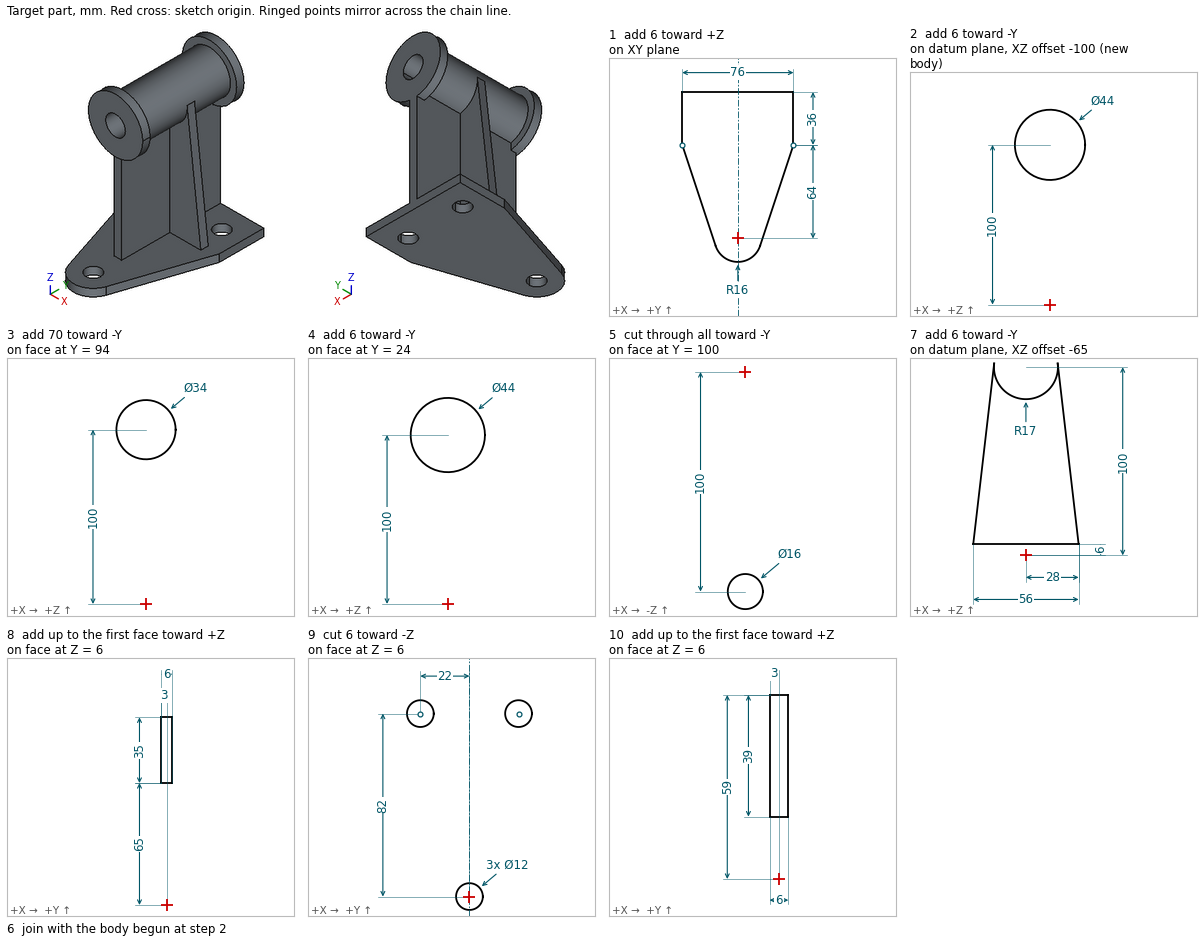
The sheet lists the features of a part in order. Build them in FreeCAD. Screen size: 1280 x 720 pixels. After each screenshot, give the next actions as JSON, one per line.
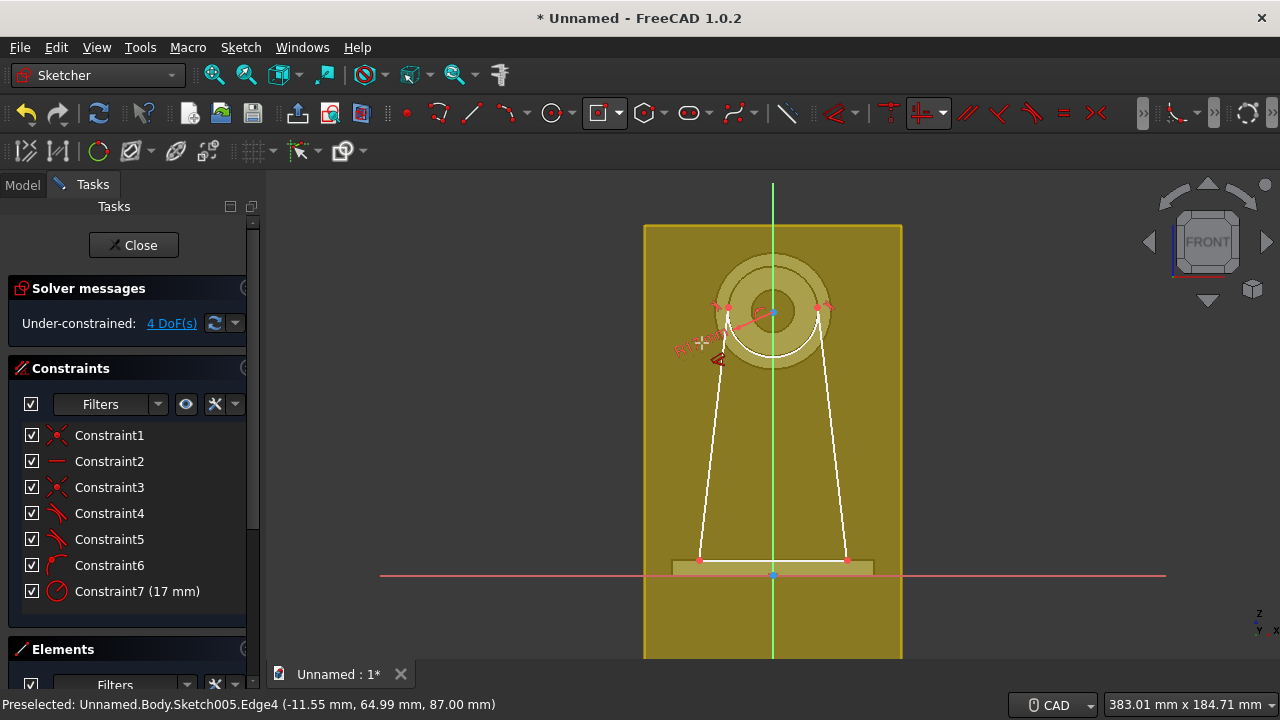
{"action": "left_click", "coordinate": [803, 561]}
{"action": "left_click", "coordinate": [739, 595]}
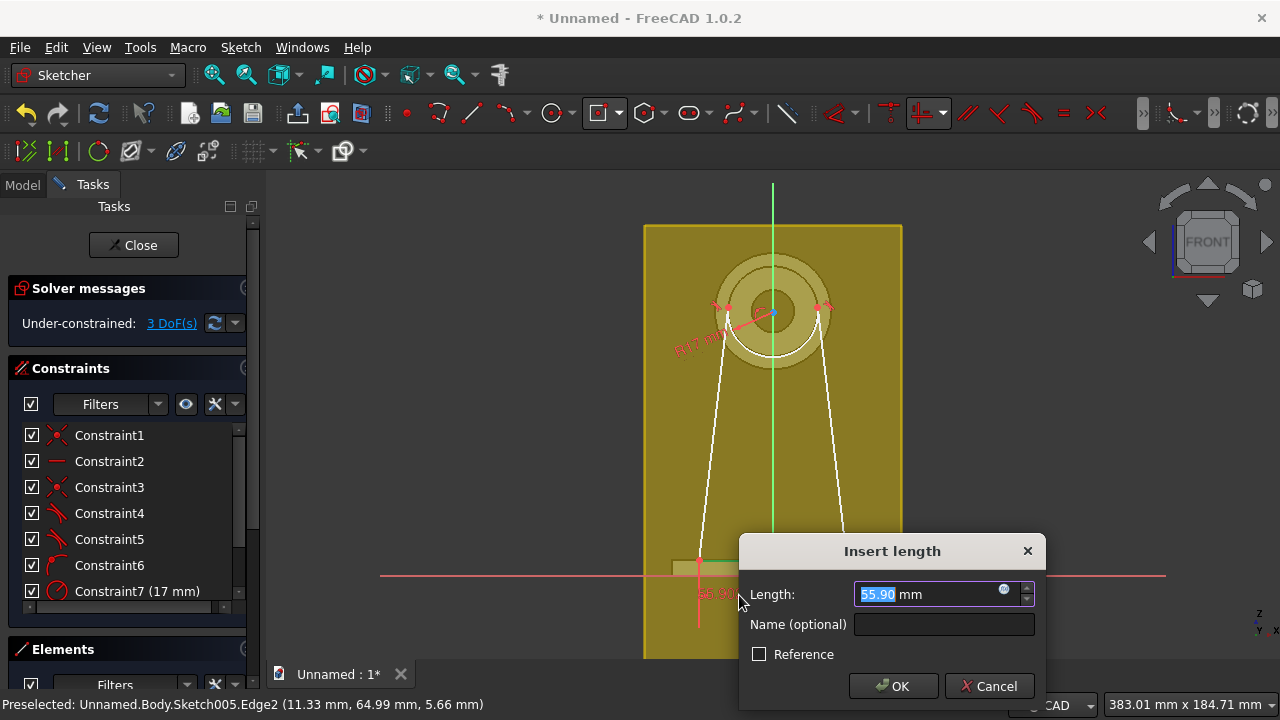
{"action": "type", "text": "56"}
{"action": "key", "text": "Return"}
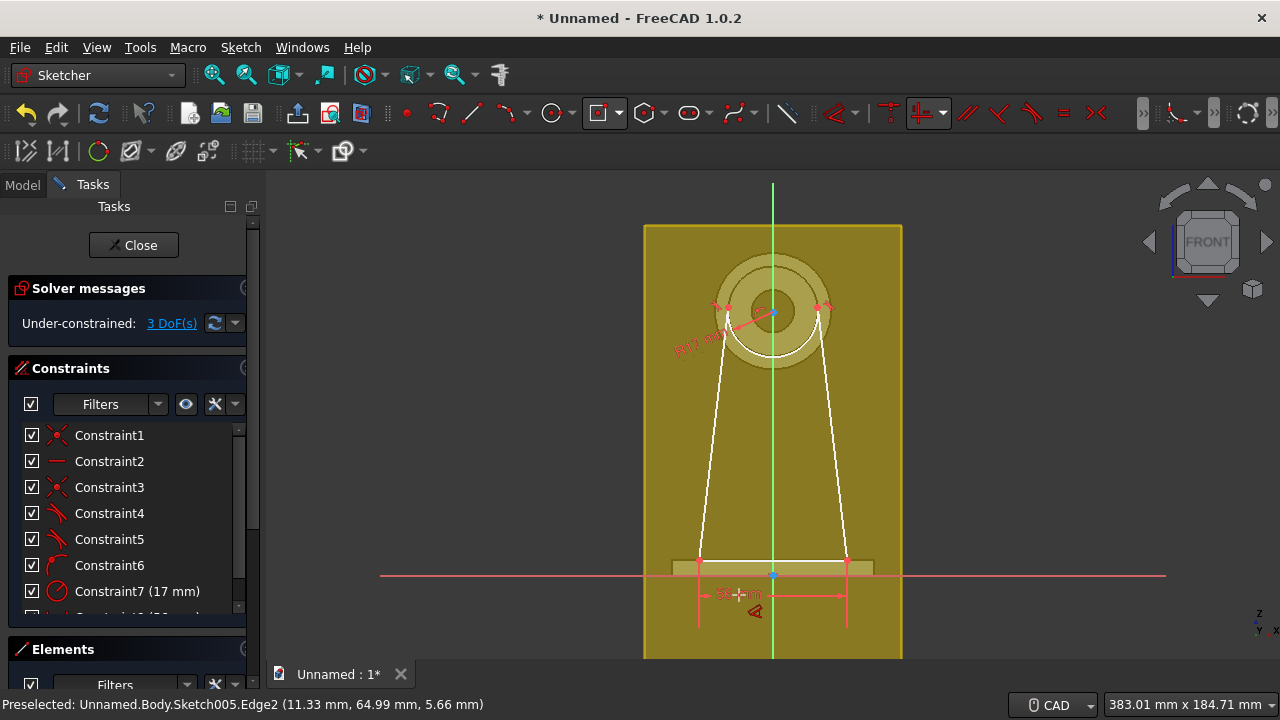
{"action": "scroll", "coordinate": [847, 561], "scroll_direction": "up", "scroll_amount": 5}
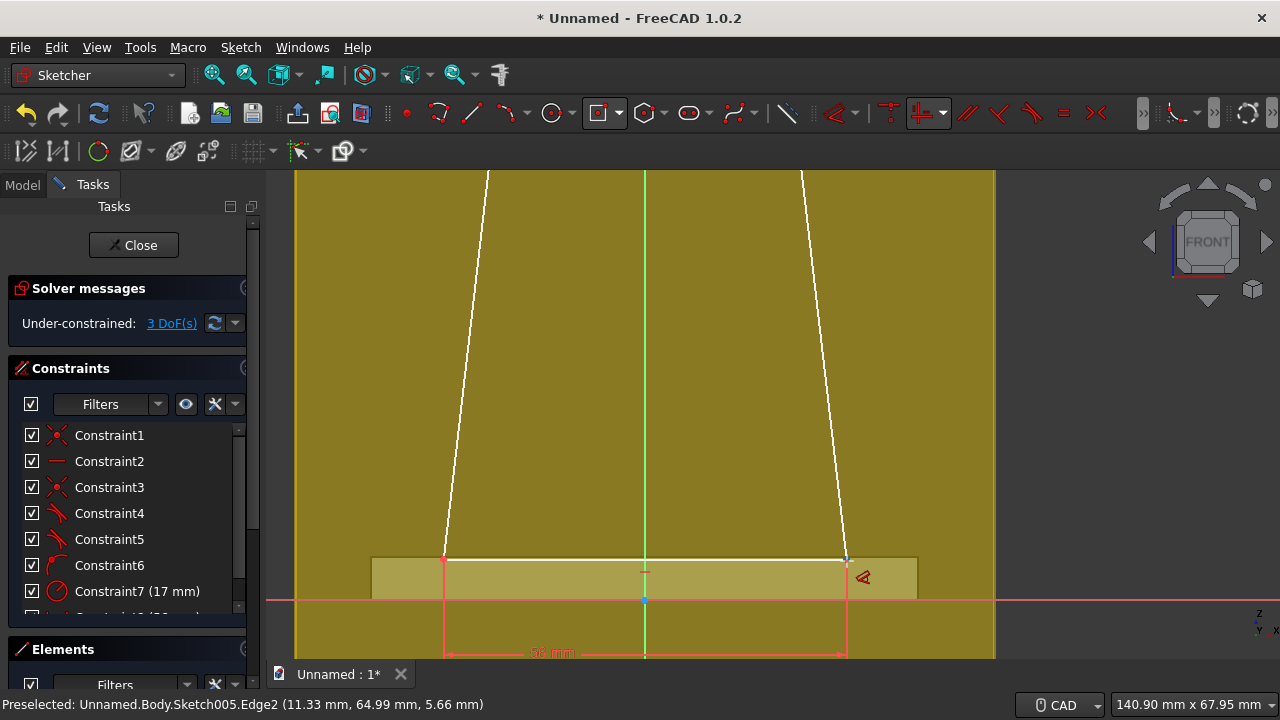
{"action": "left_click", "coordinate": [847, 560]}
{"action": "left_click", "coordinate": [881, 580]}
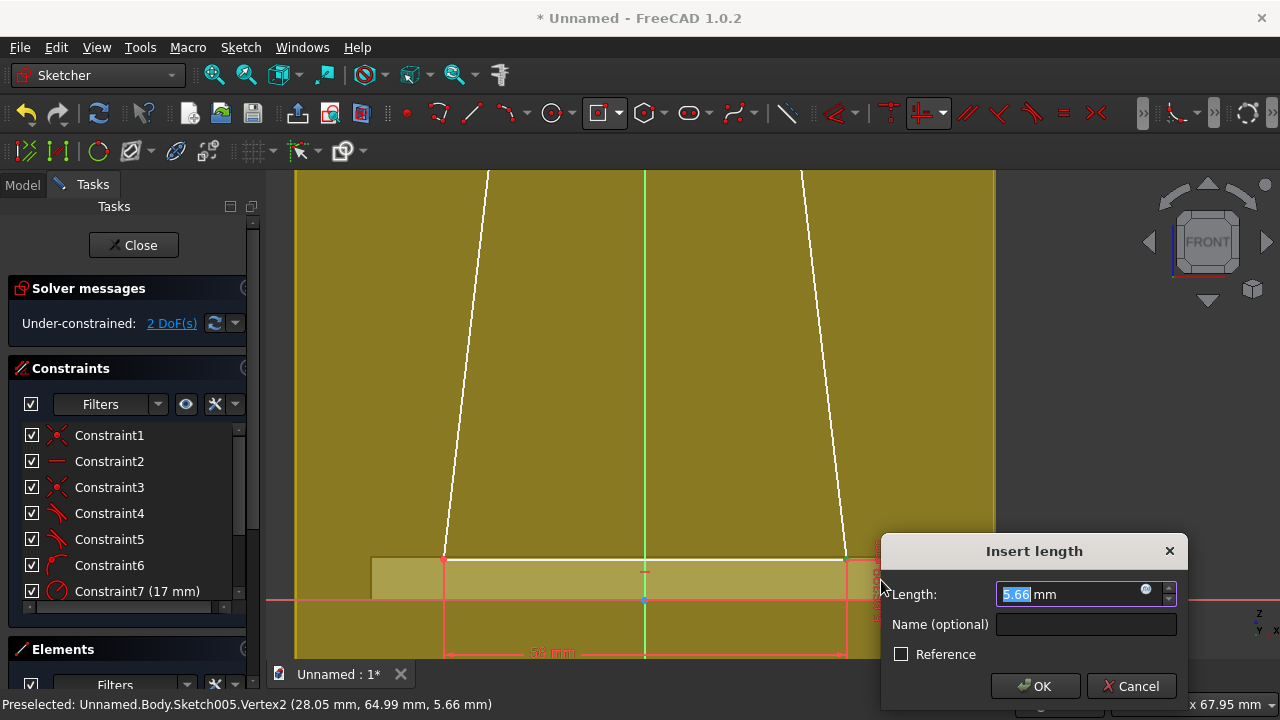
{"action": "type", "text": "6"}
{"action": "key", "text": "Return"}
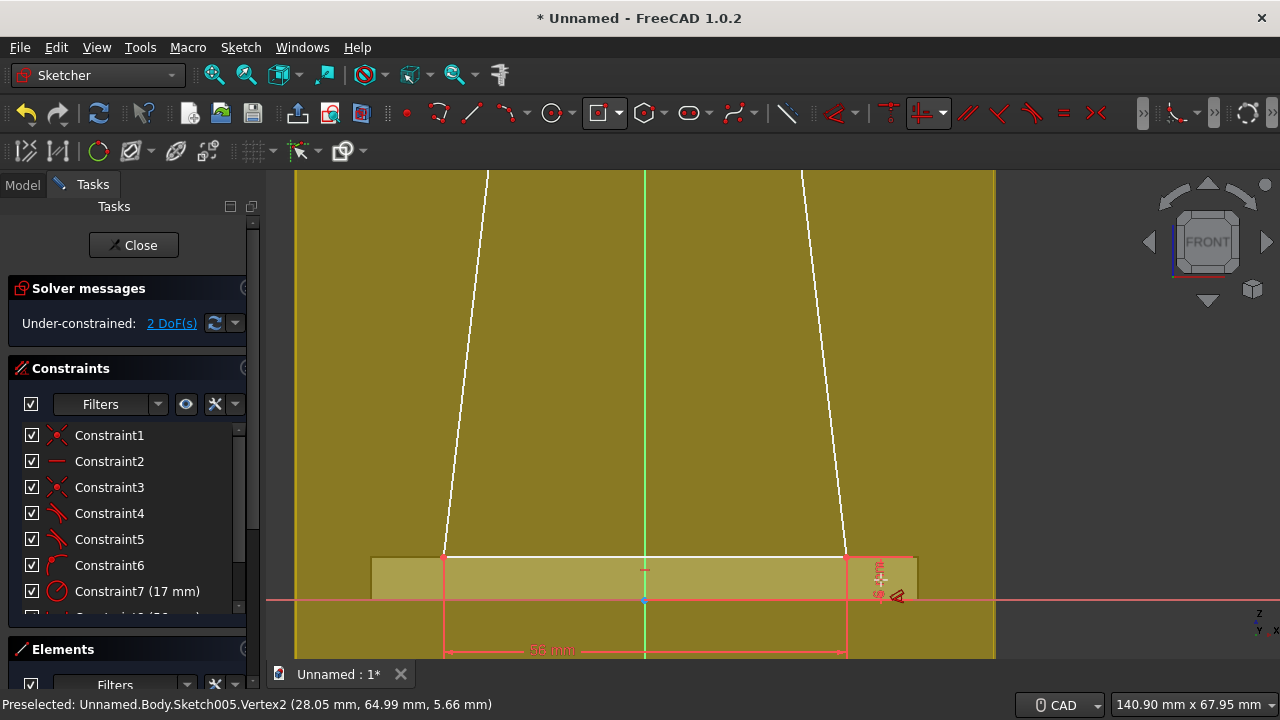
{"action": "left_click", "coordinate": [847, 557]}
{"action": "left_click", "coordinate": [746, 523]}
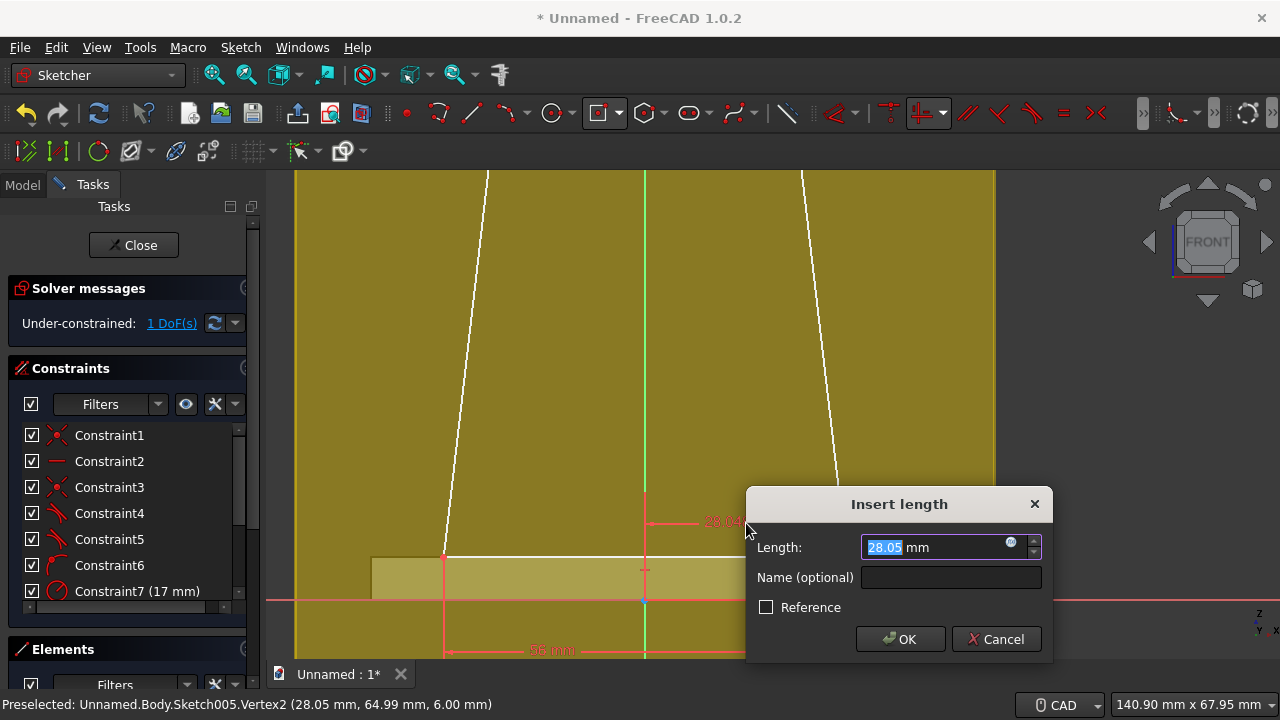
{"action": "type", "text": "28"}
{"action": "key", "text": "Return"}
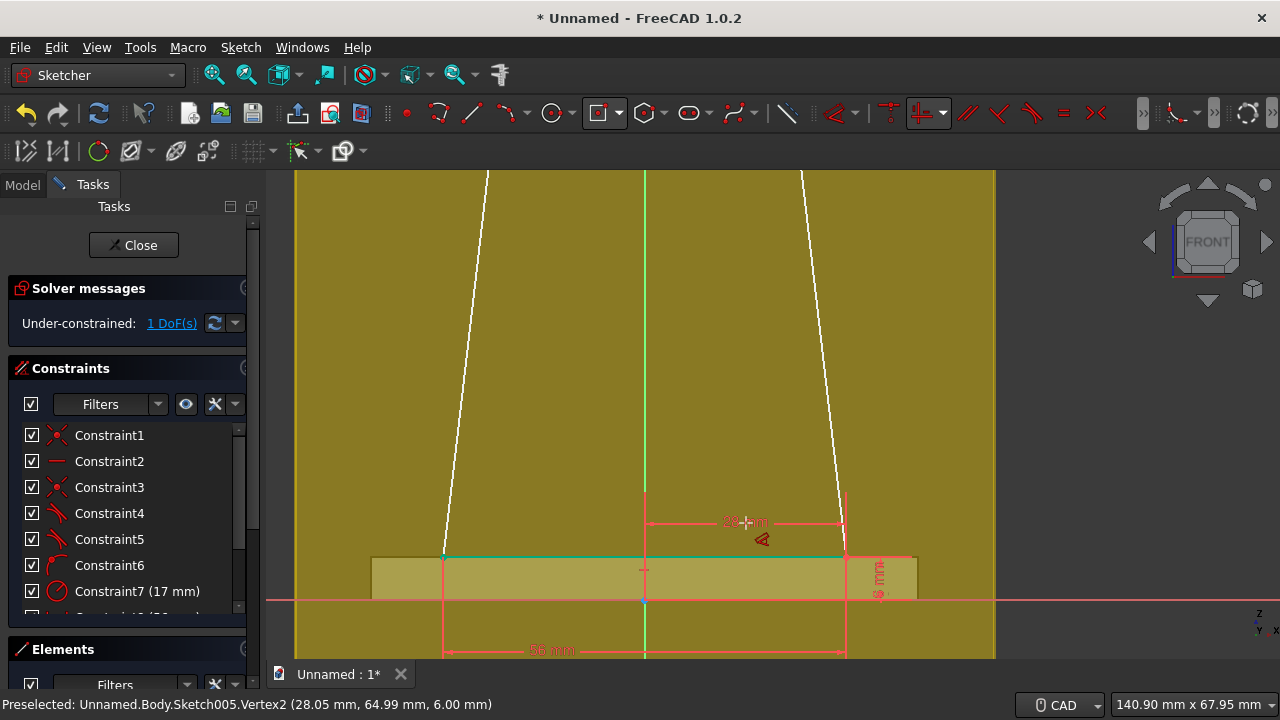
{"action": "scroll", "coordinate": [753, 562], "scroll_direction": "down", "scroll_amount": 4}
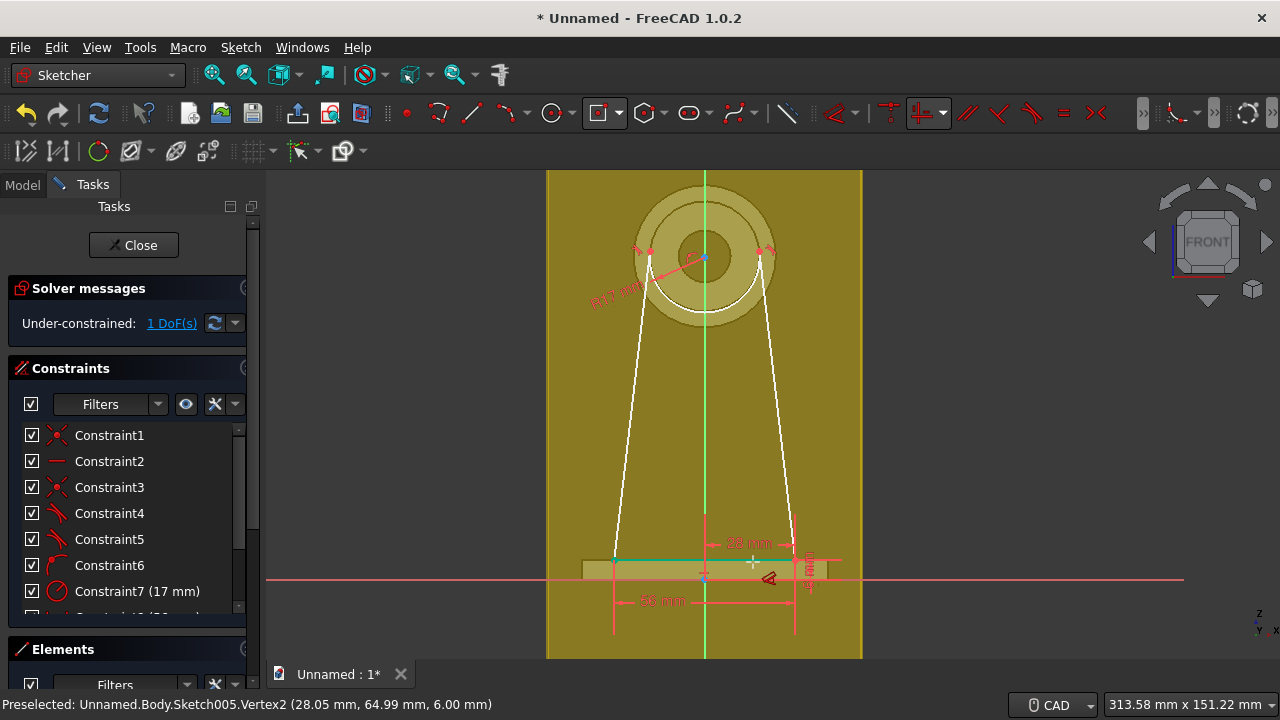
{"action": "left_click", "coordinate": [705, 258]}
{"action": "left_click", "coordinate": [739, 419]}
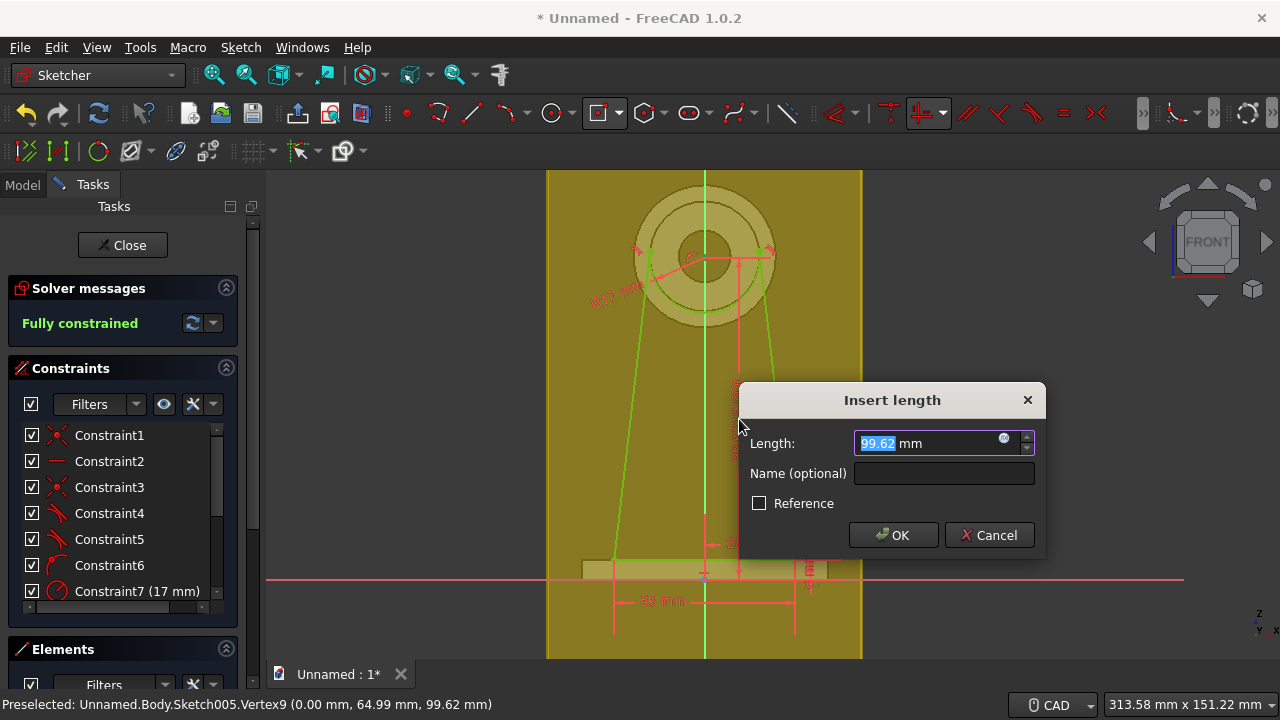
{"action": "type", "text": "100"}
{"action": "key", "text": "Return"}
{"action": "key", "text": "Escape"}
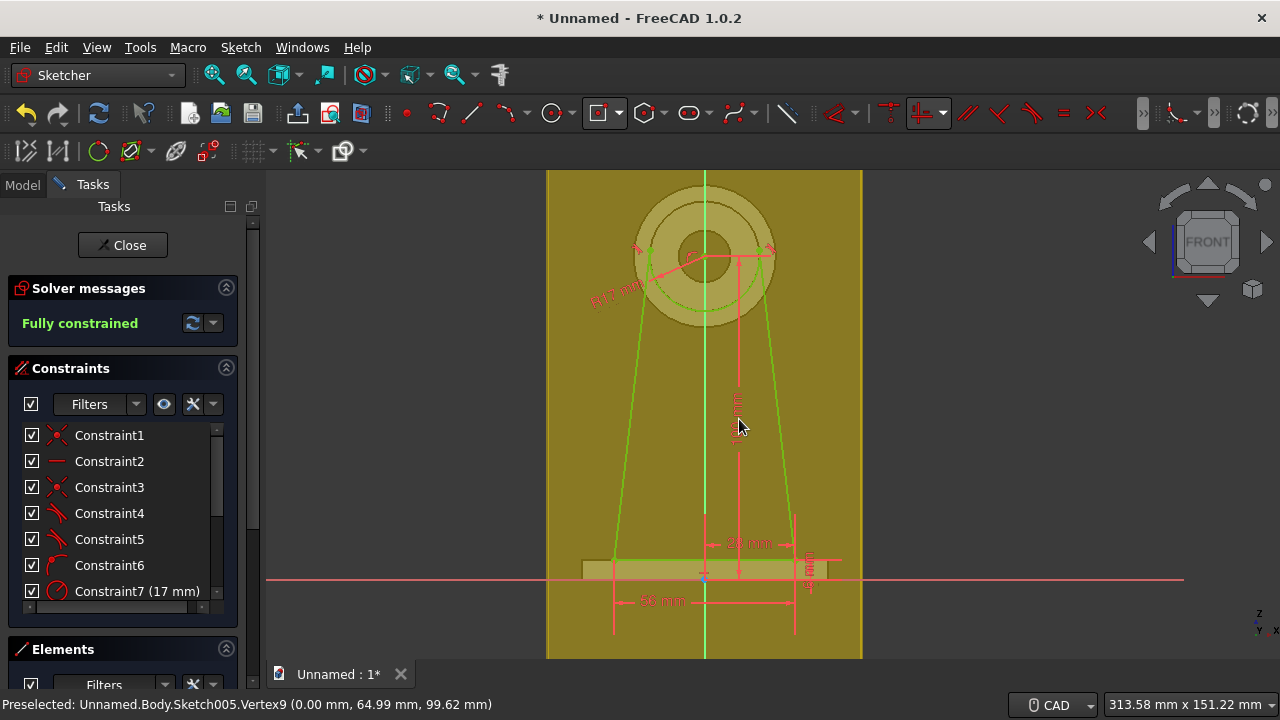
{"action": "left_click", "coordinate": [123, 245]}